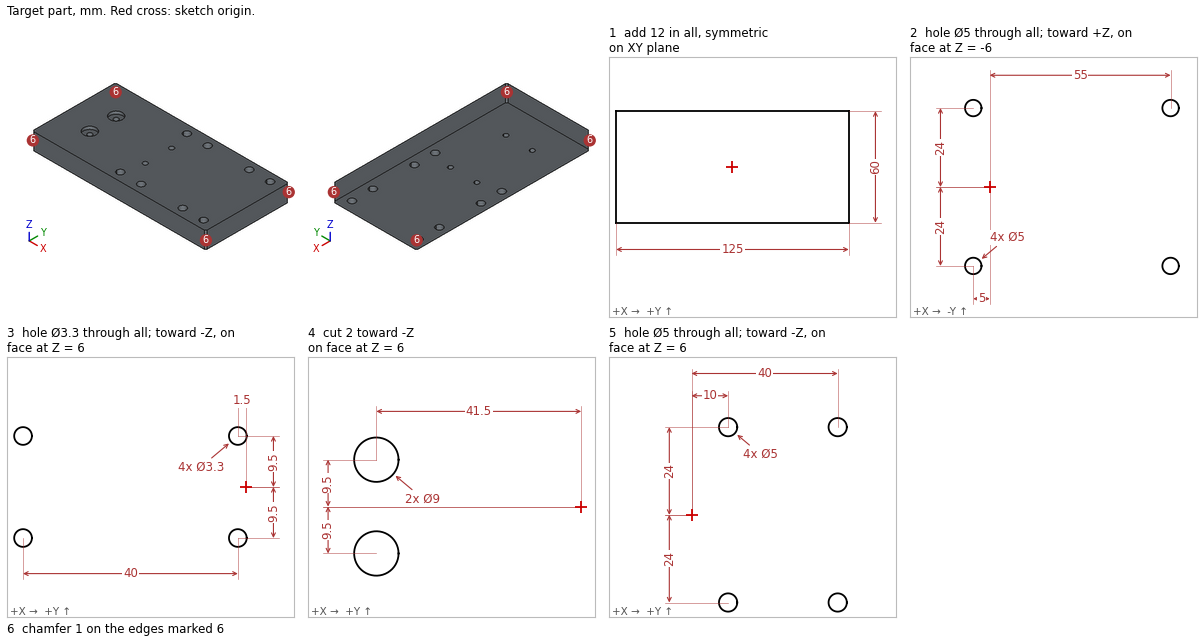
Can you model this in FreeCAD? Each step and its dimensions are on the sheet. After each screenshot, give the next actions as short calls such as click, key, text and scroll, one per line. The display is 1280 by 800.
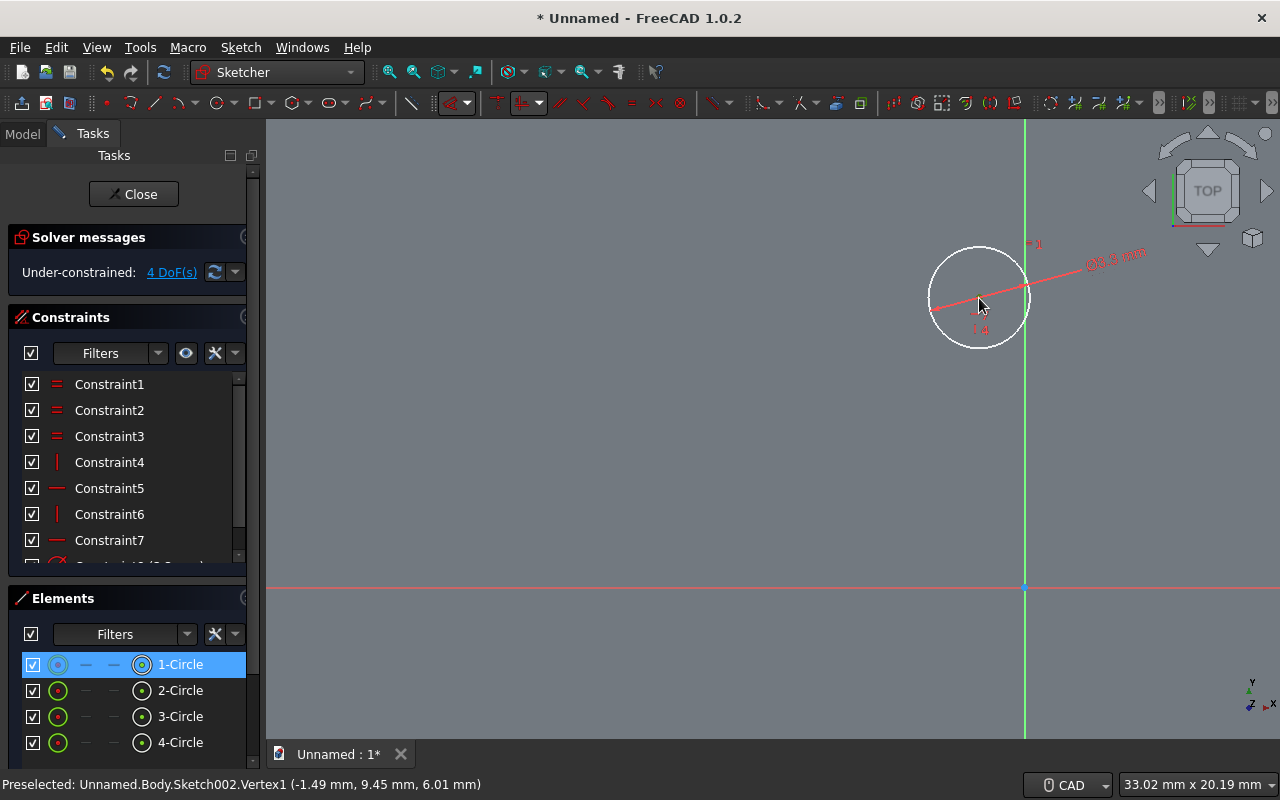
key(l)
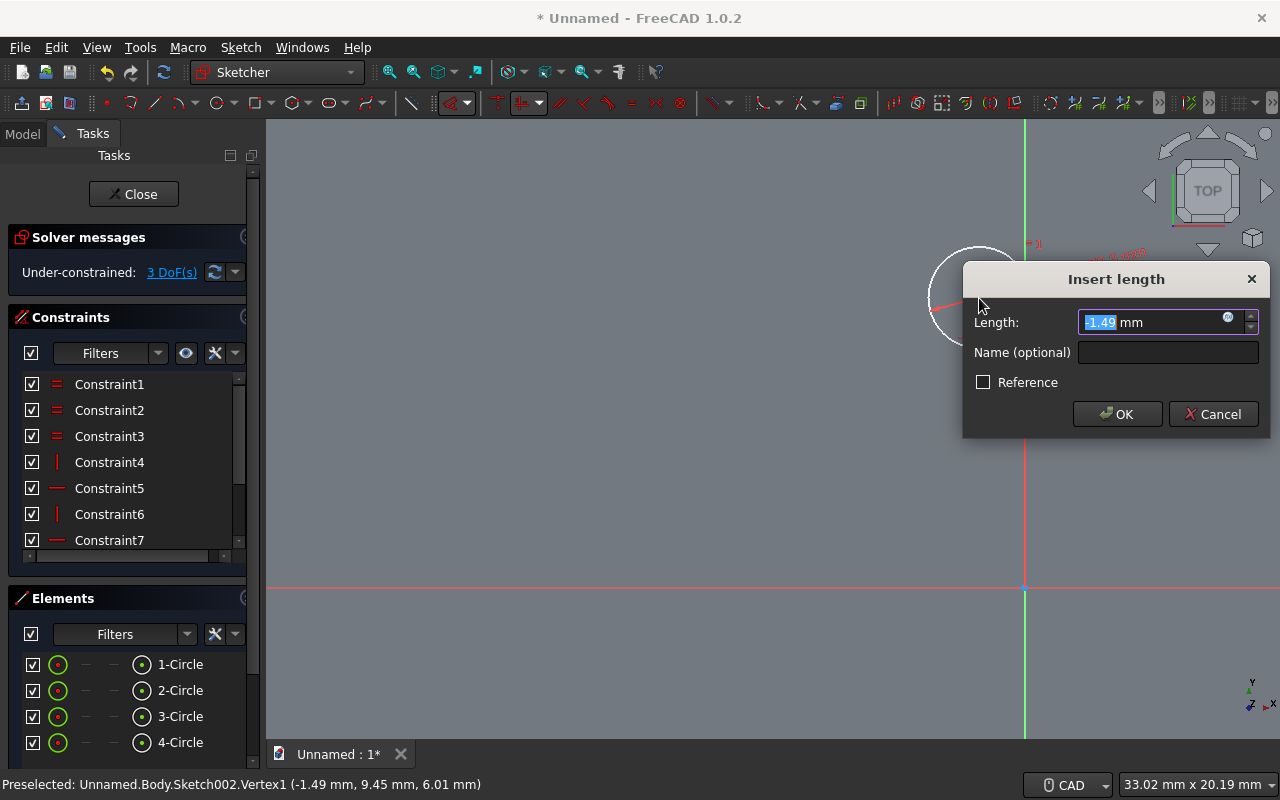
text(-1.5)
key(Return)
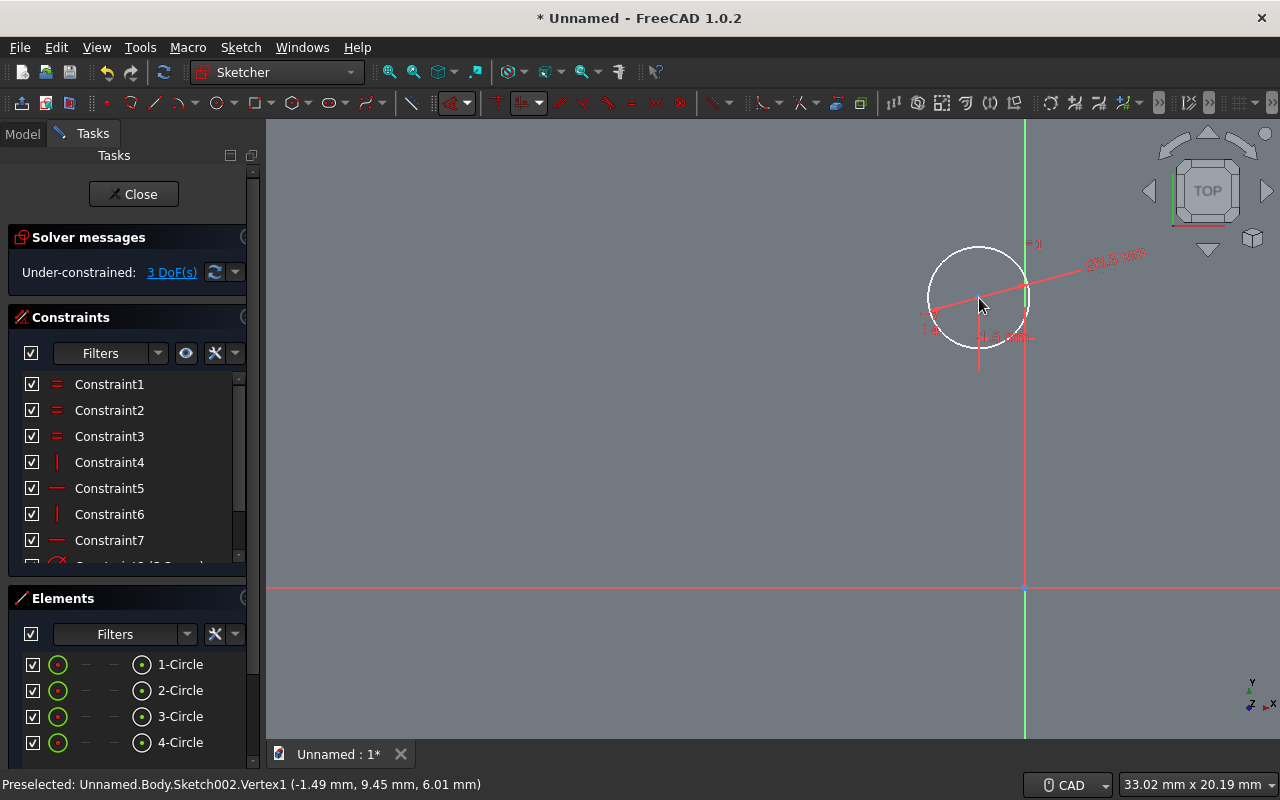
click(979, 298)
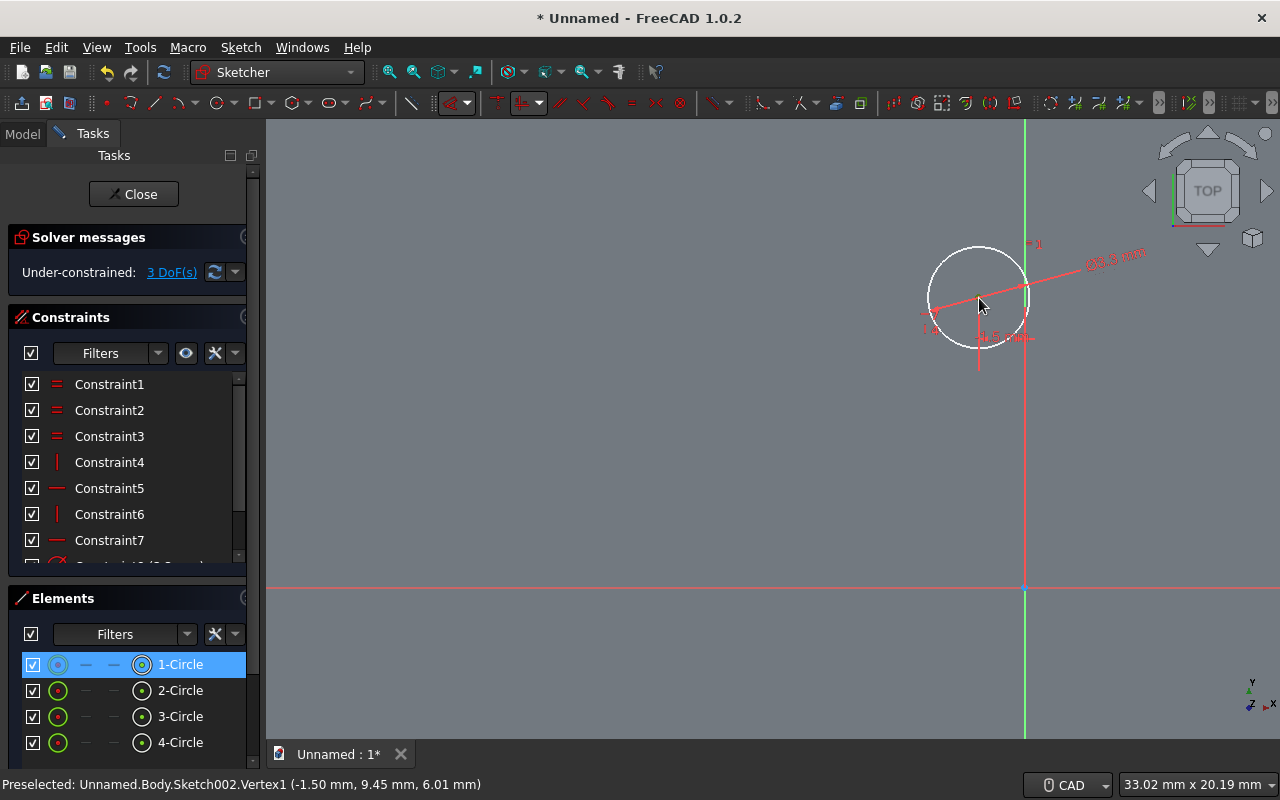
click(470, 104)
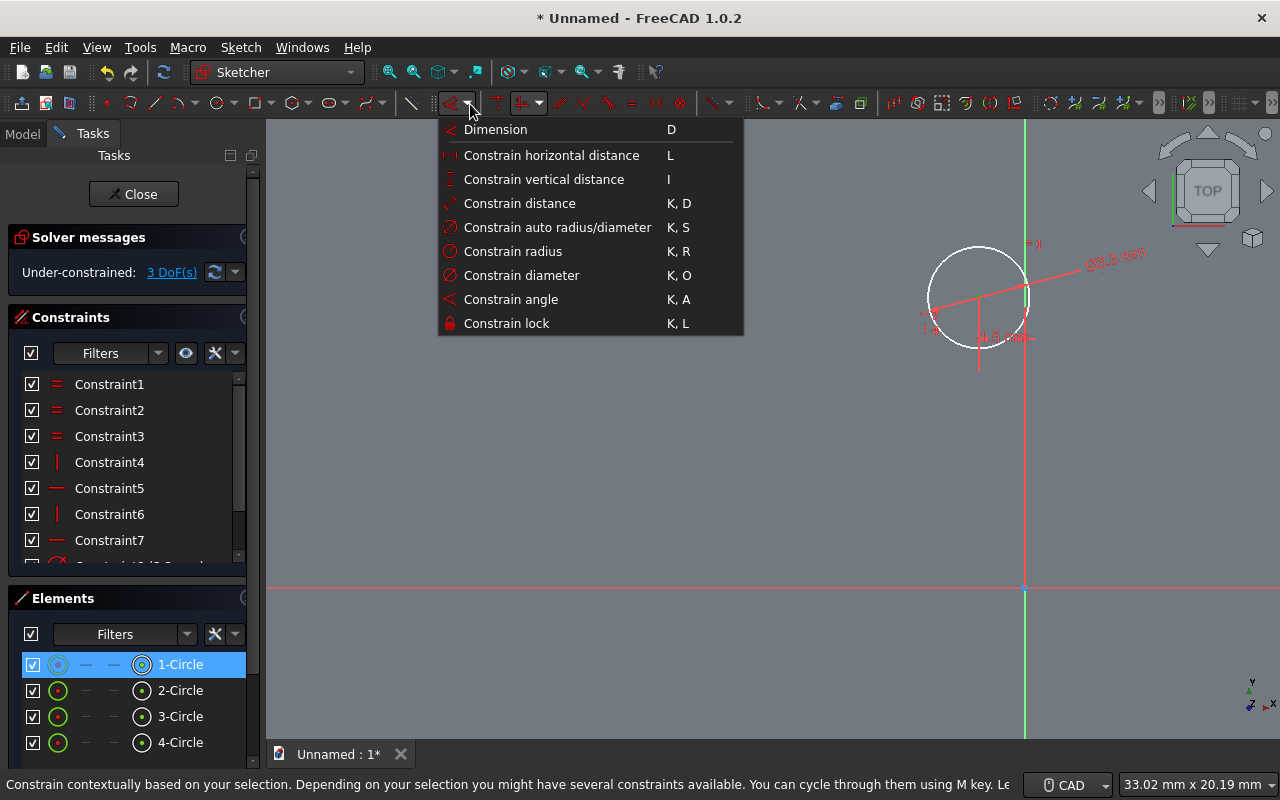
click(591, 179)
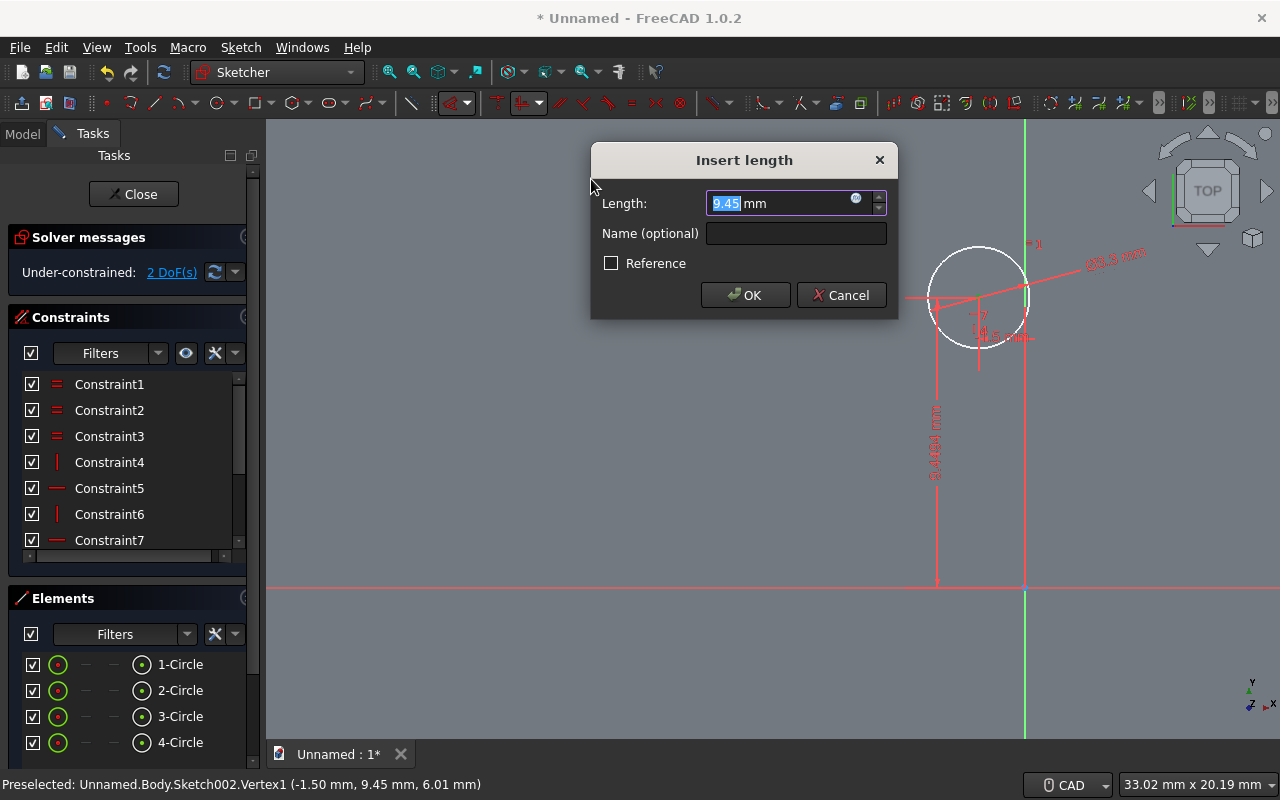
text(9.5)
key(Return)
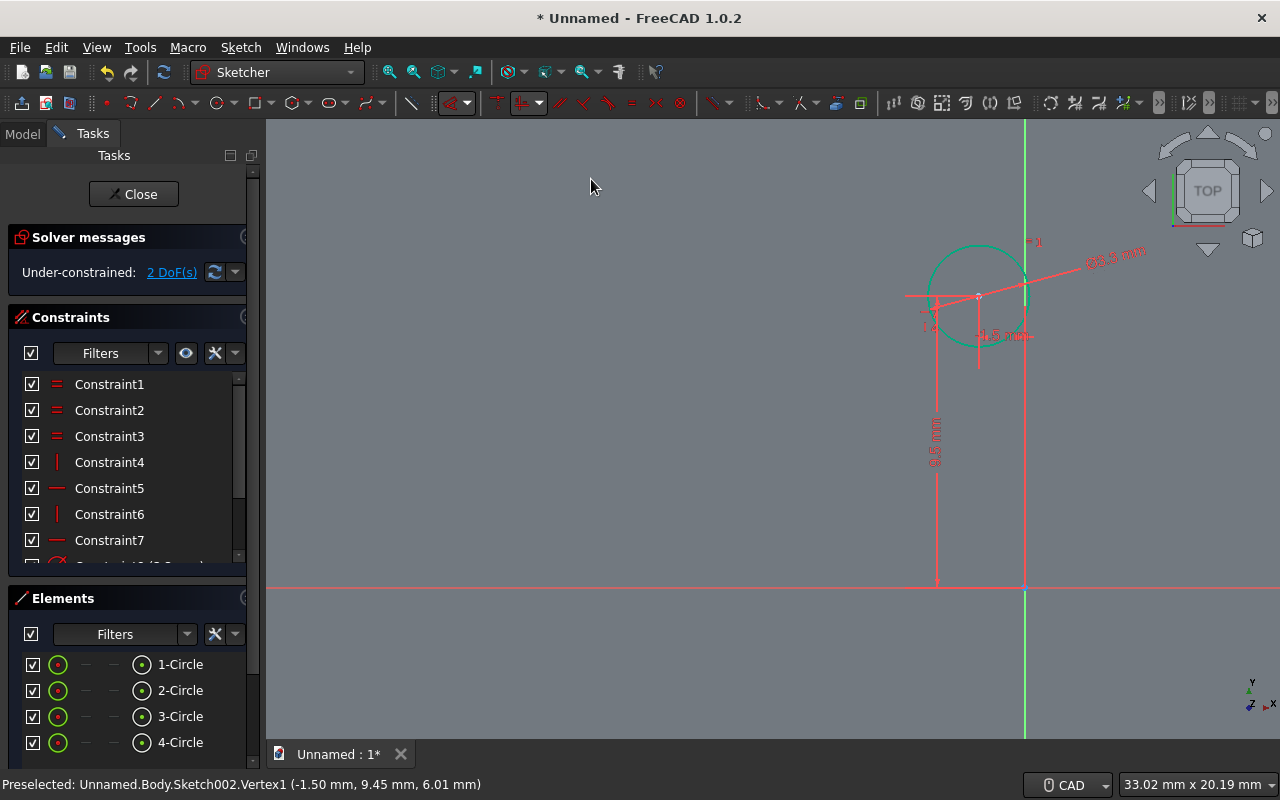
scroll(982, 299, down, 4)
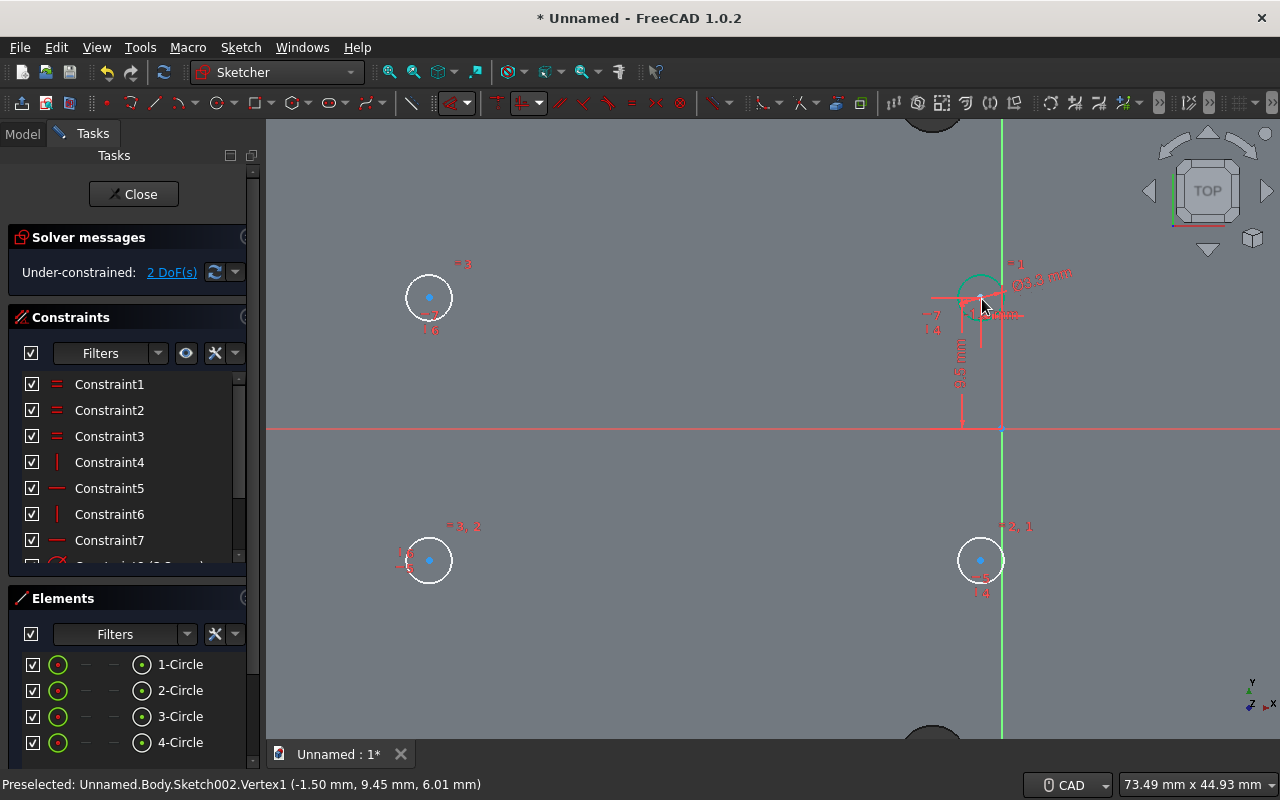
click(981, 561)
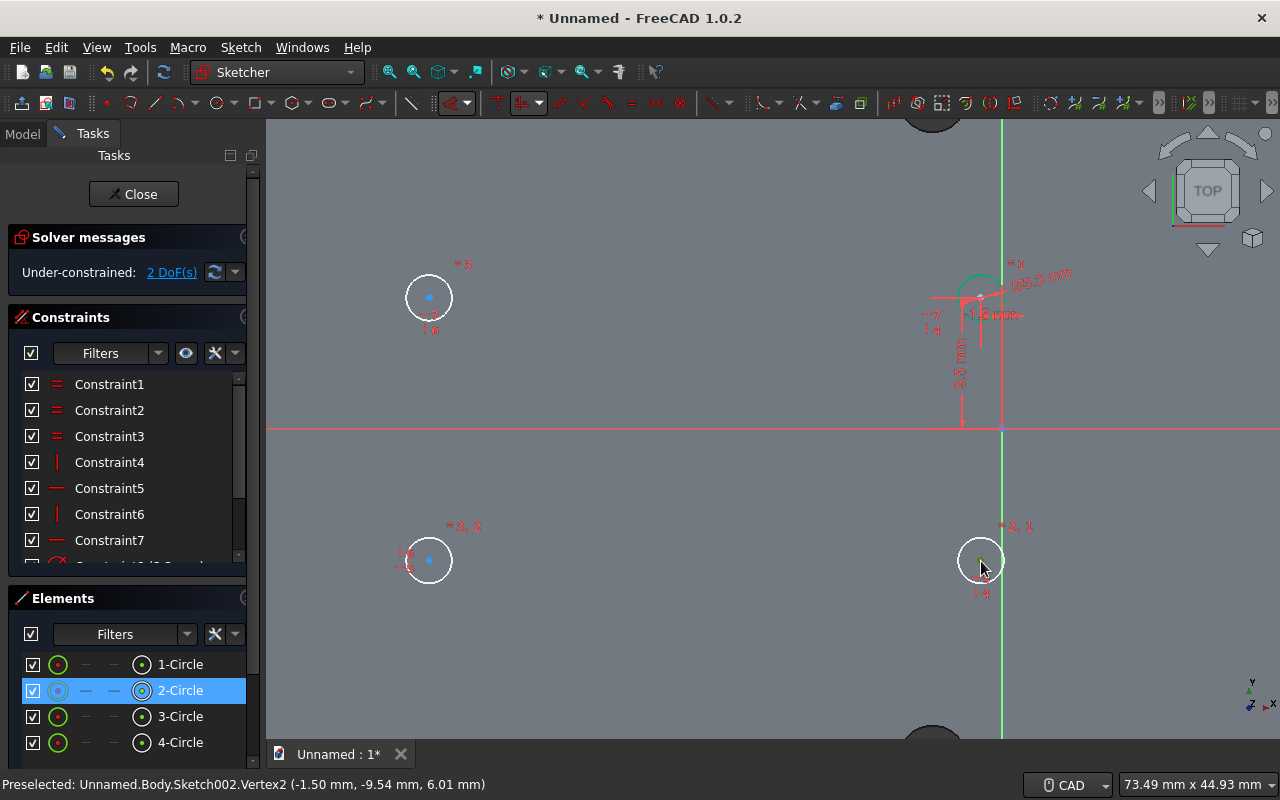
key(i)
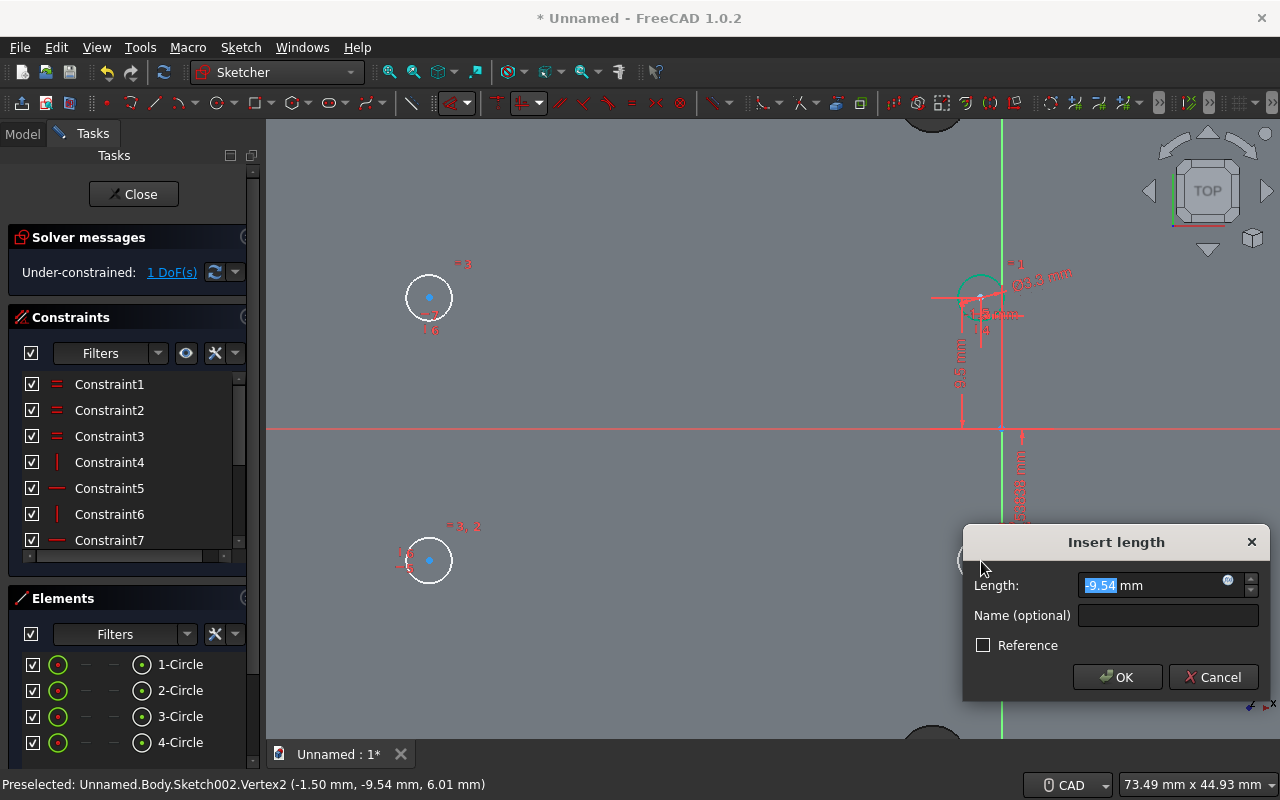
text(-9.5)
key(Return)